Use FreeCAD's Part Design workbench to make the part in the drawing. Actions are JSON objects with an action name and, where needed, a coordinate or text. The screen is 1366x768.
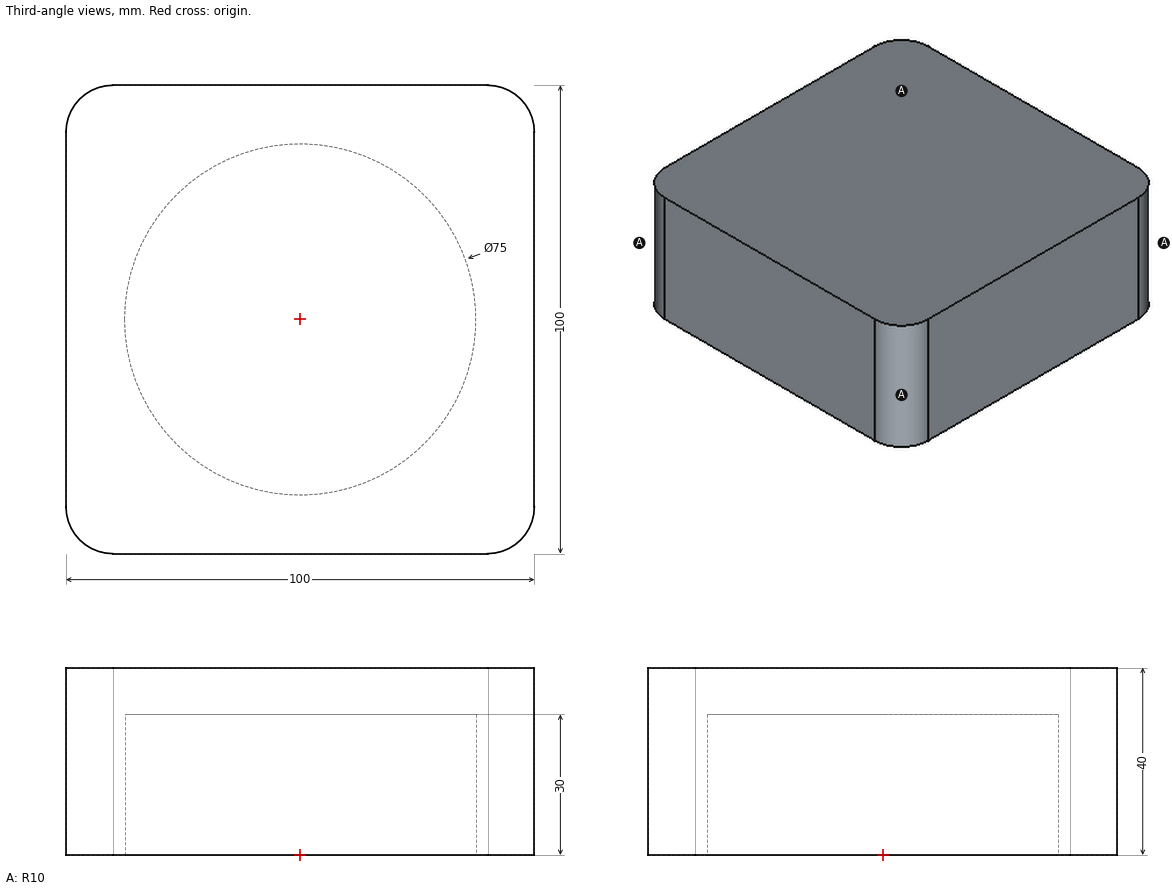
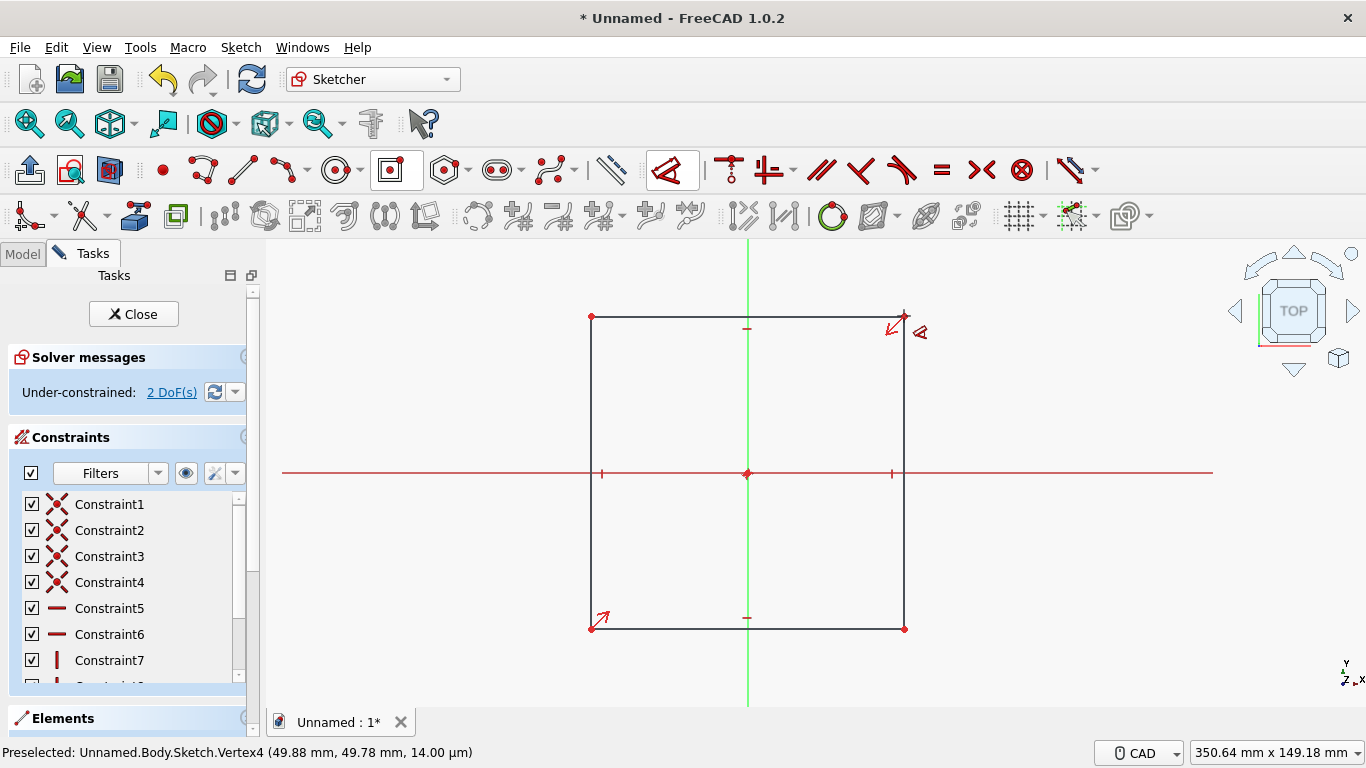
{"action": "left_click", "coordinate": [685, 629]}
{"action": "left_click", "coordinate": [676, 663]}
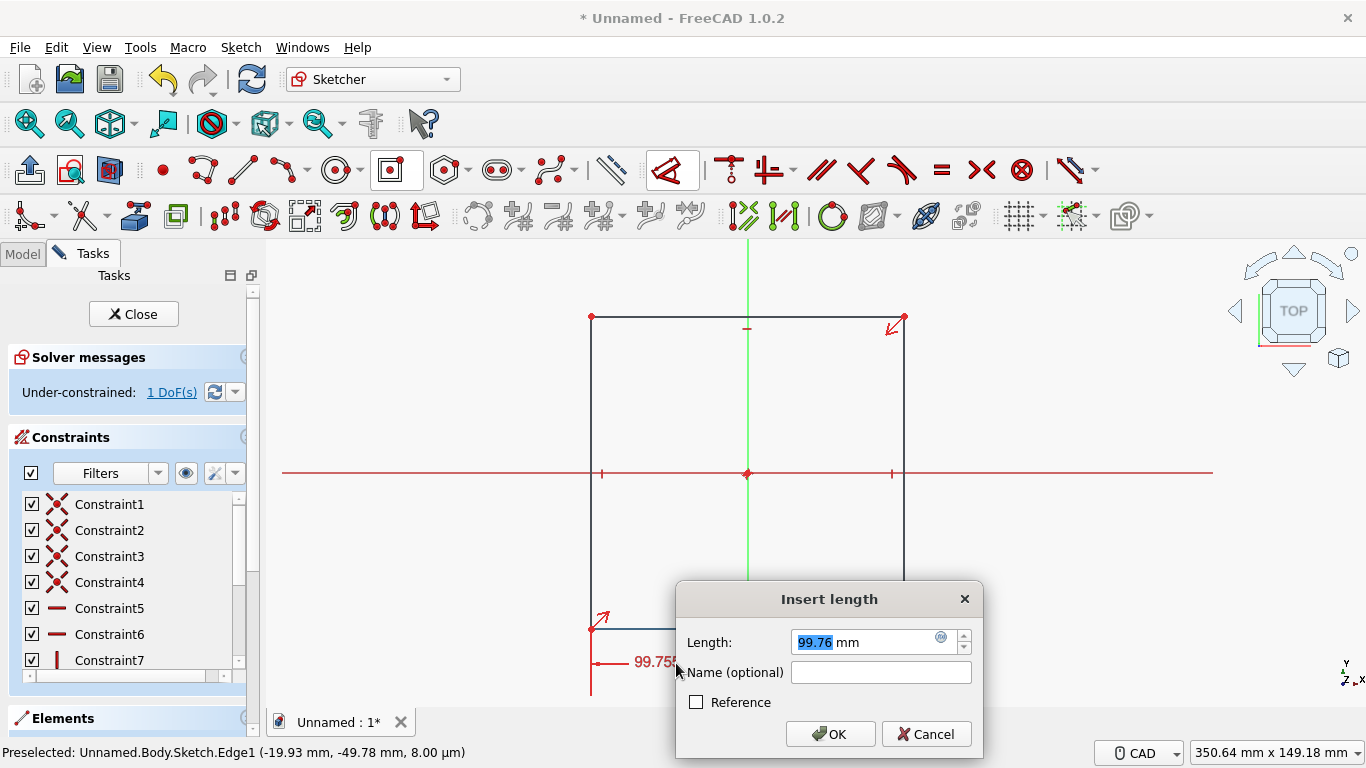
{"action": "type", "text": "100"}
{"action": "key", "text": "Return"}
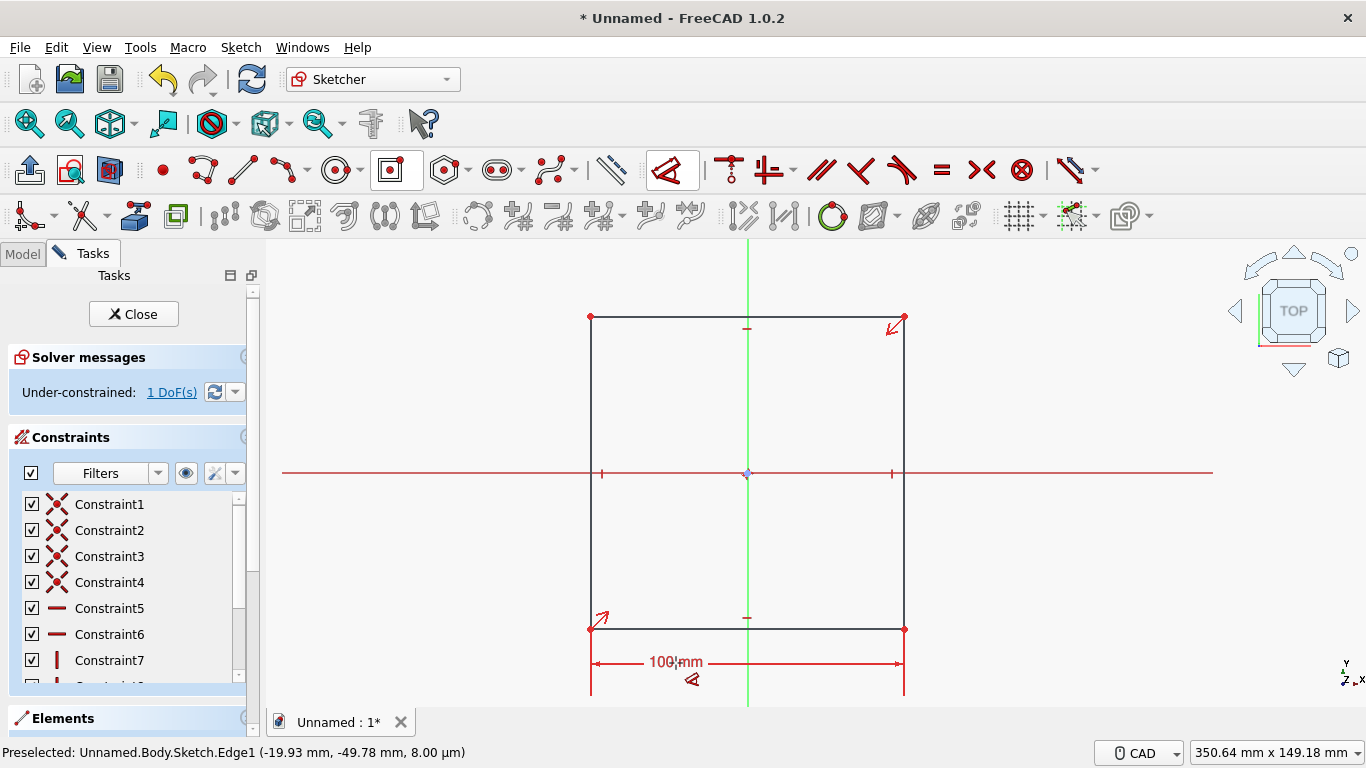
{"action": "left_click", "coordinate": [904, 536]}
{"action": "left_click", "coordinate": [938, 401]}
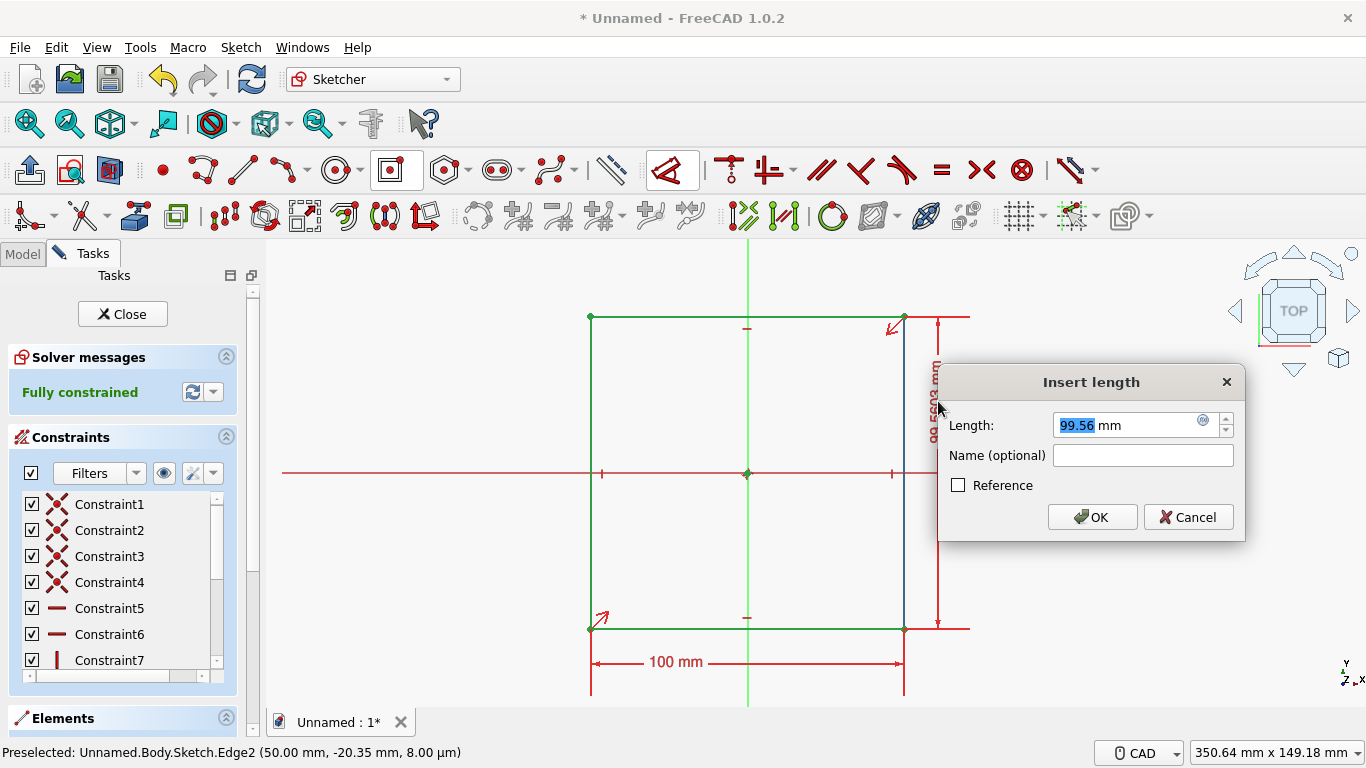
{"action": "type", "text": "100"}
{"action": "key", "text": "Return"}
{"action": "key", "text": "Escape"}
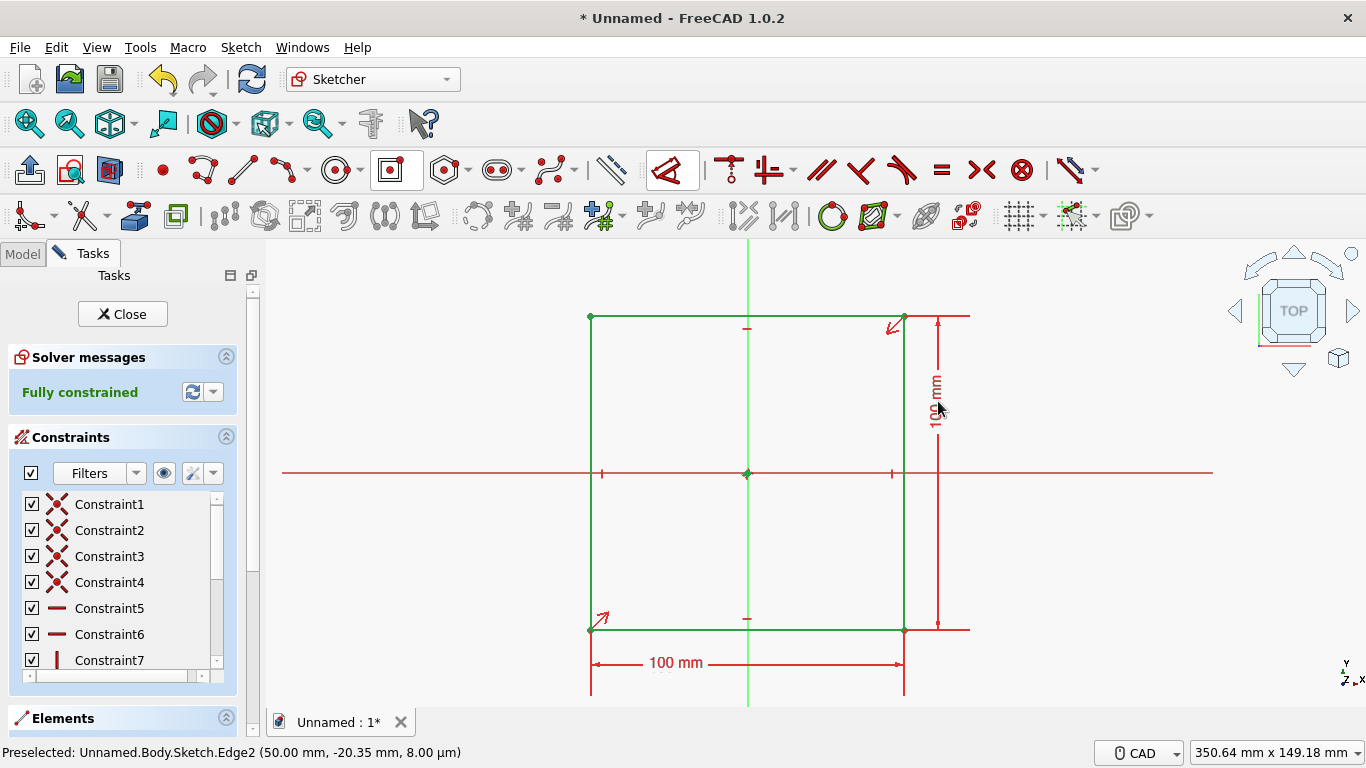
{"action": "left_click", "coordinate": [123, 314]}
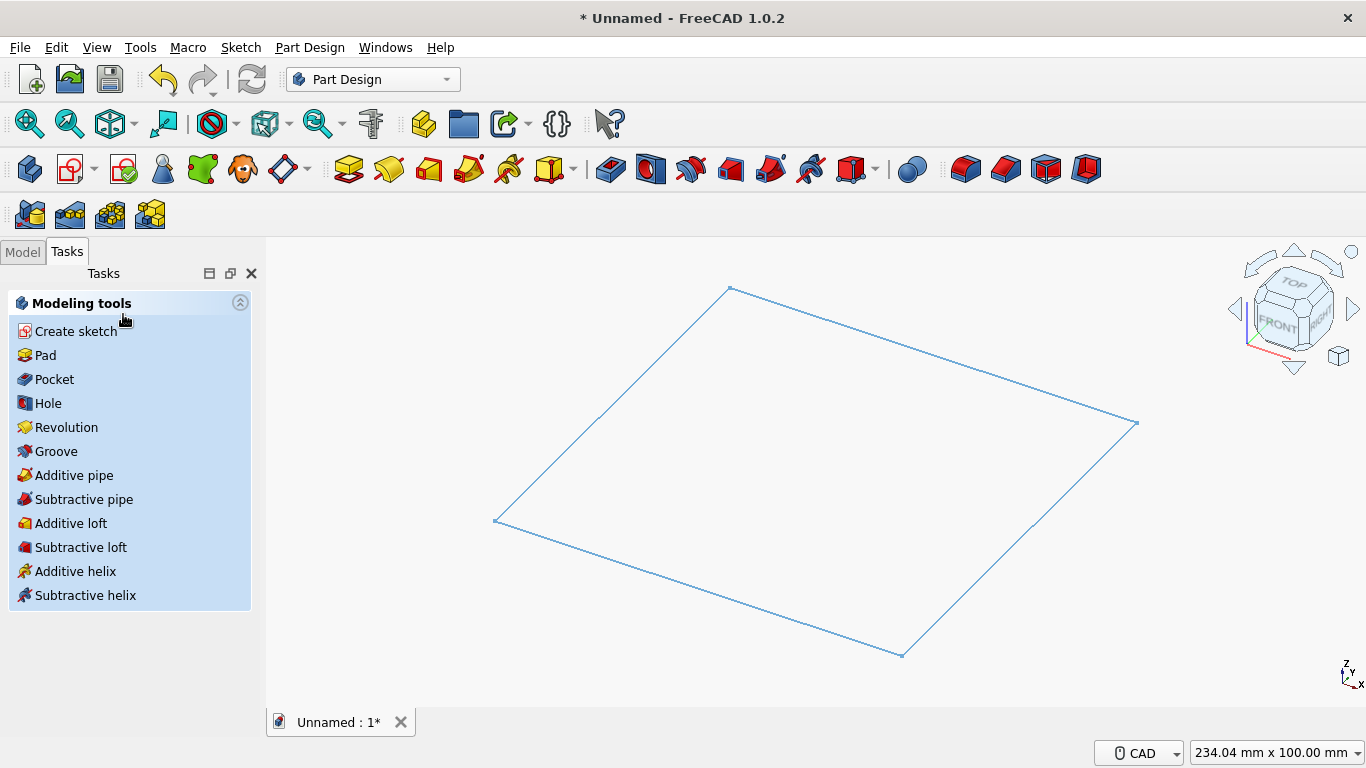
{"action": "left_click", "coordinate": [350, 170]}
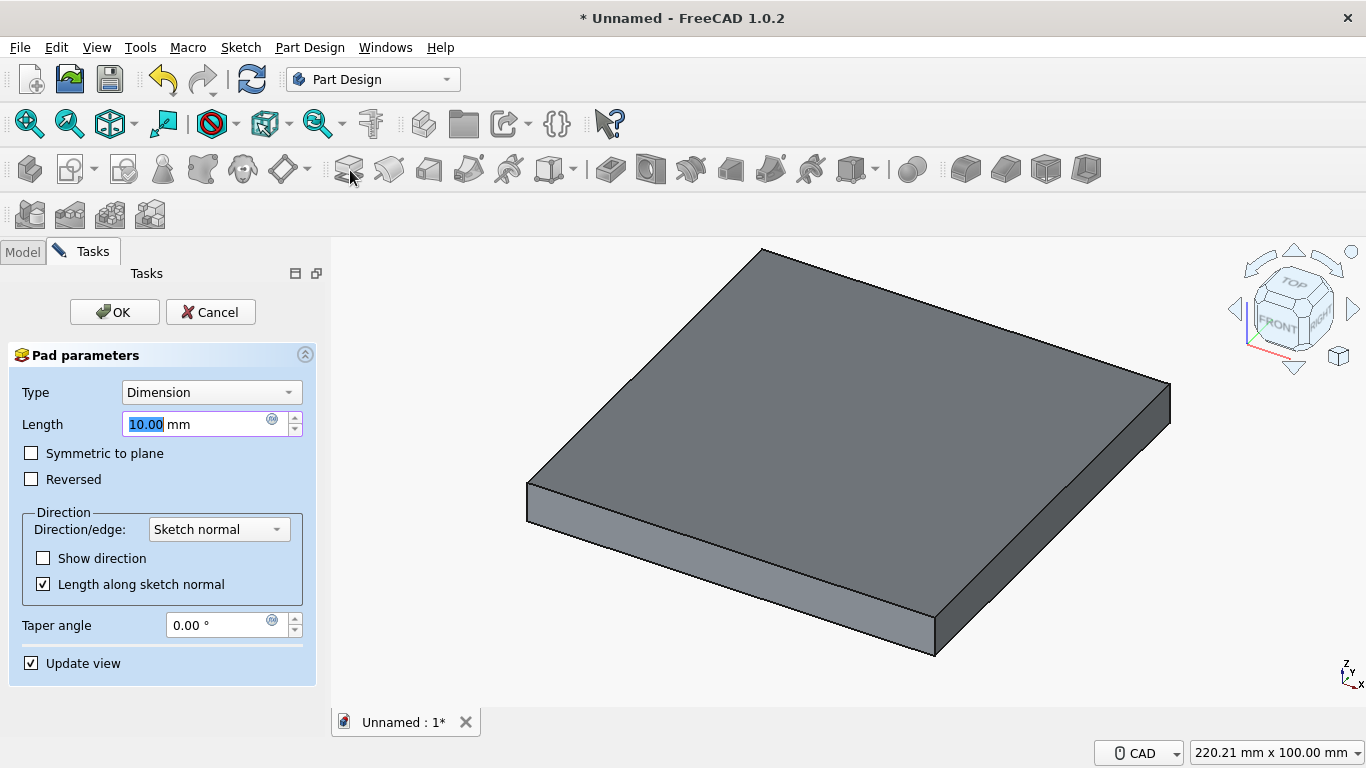
{"action": "type", "text": "40"}
{"action": "key", "text": "Tab"}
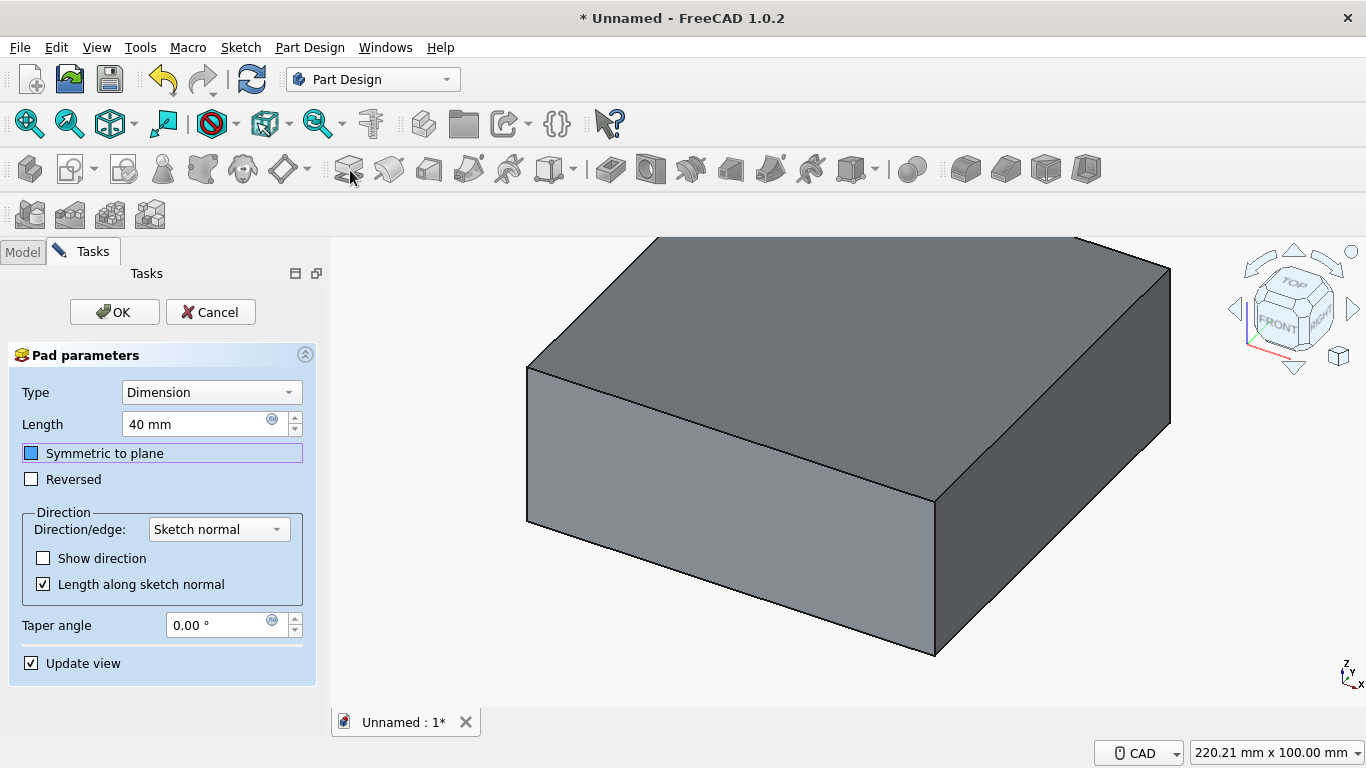
{"action": "left_click", "coordinate": [115, 312]}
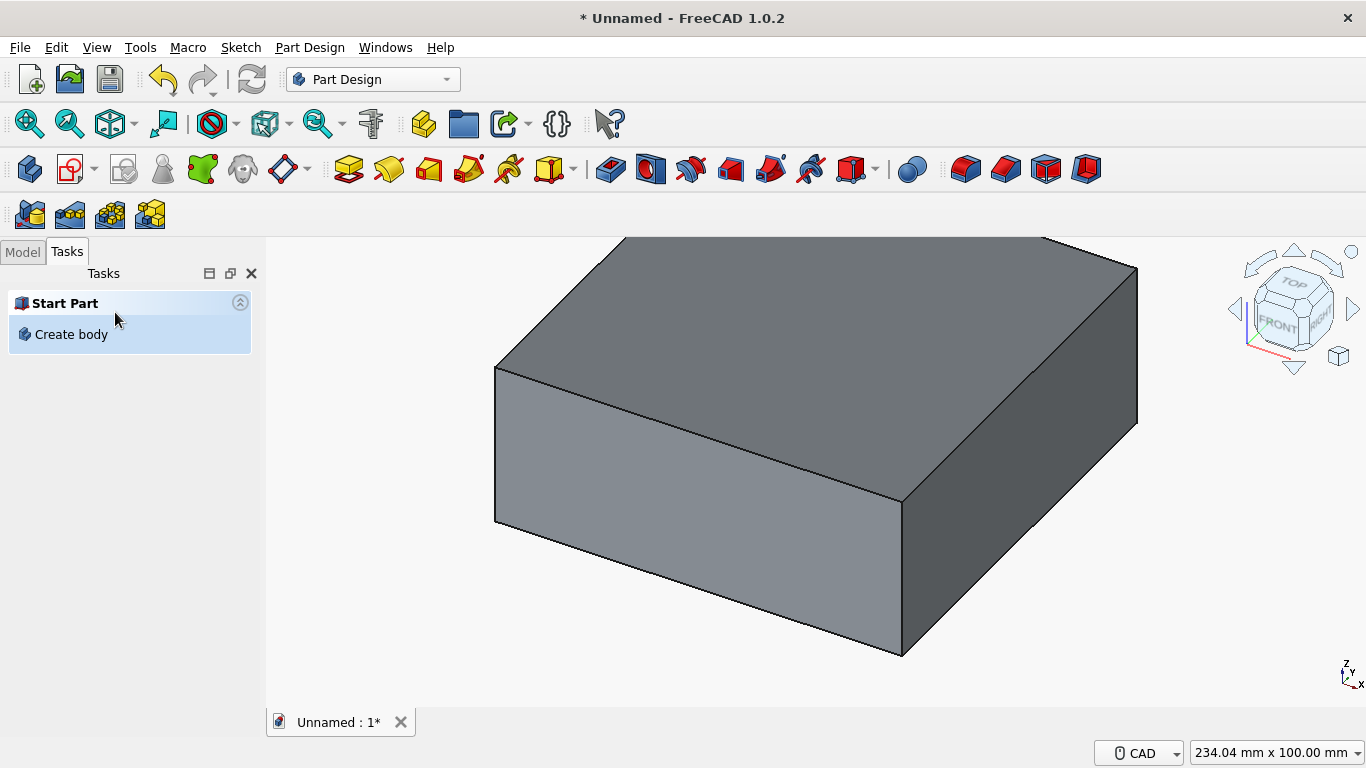
{"action": "left_click", "coordinate": [30, 124]}